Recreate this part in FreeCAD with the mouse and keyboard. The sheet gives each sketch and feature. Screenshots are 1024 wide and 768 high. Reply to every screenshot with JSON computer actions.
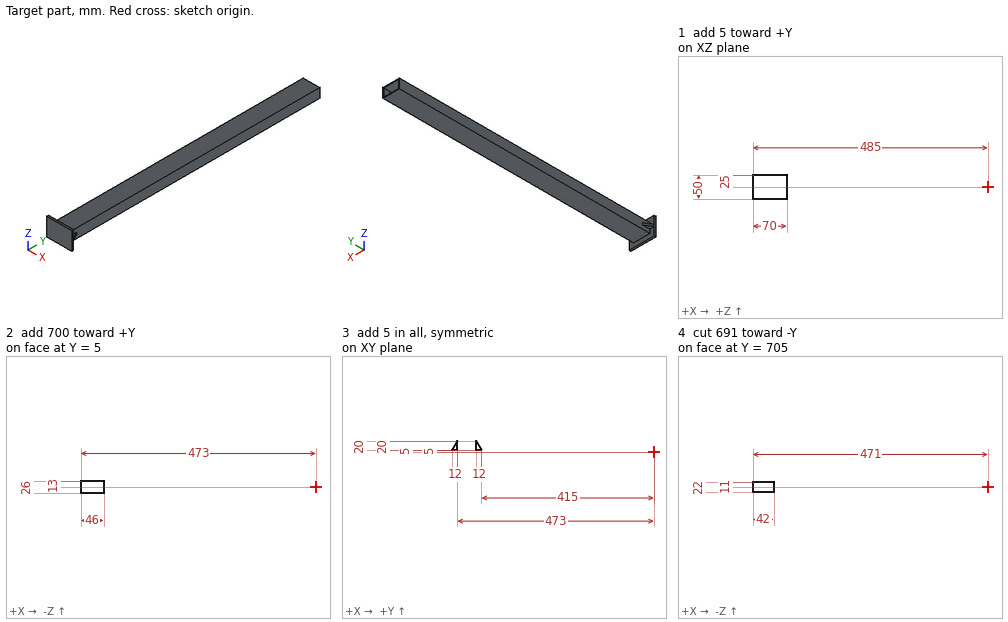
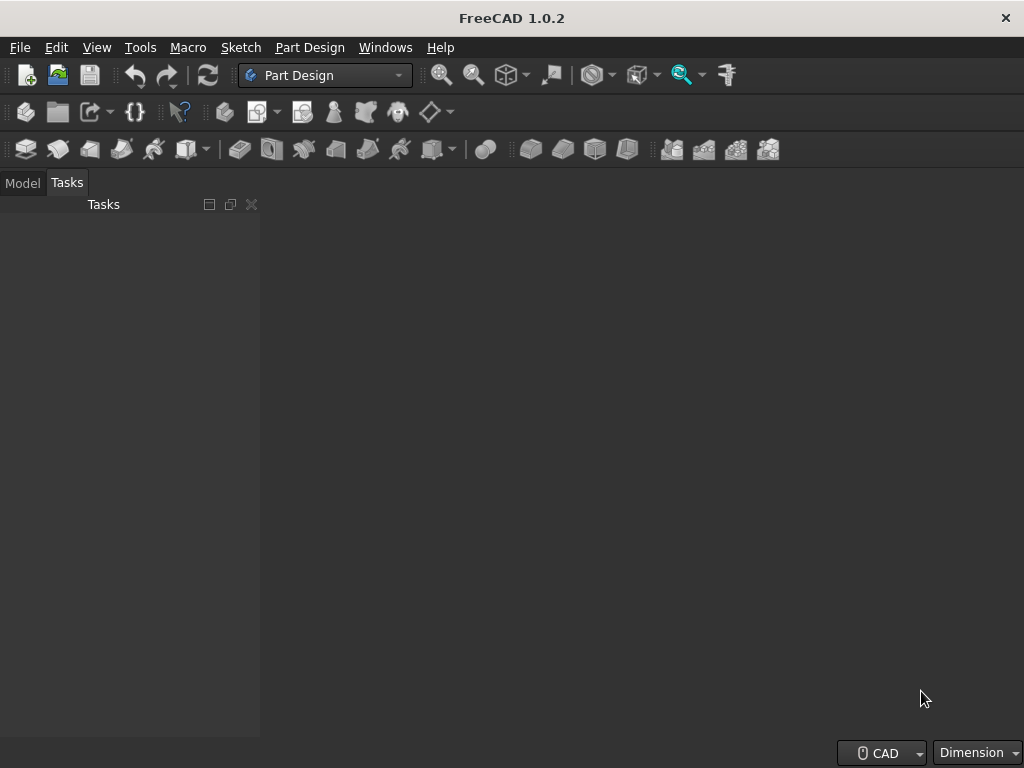
{"action": "left_click", "coordinate": [26, 76]}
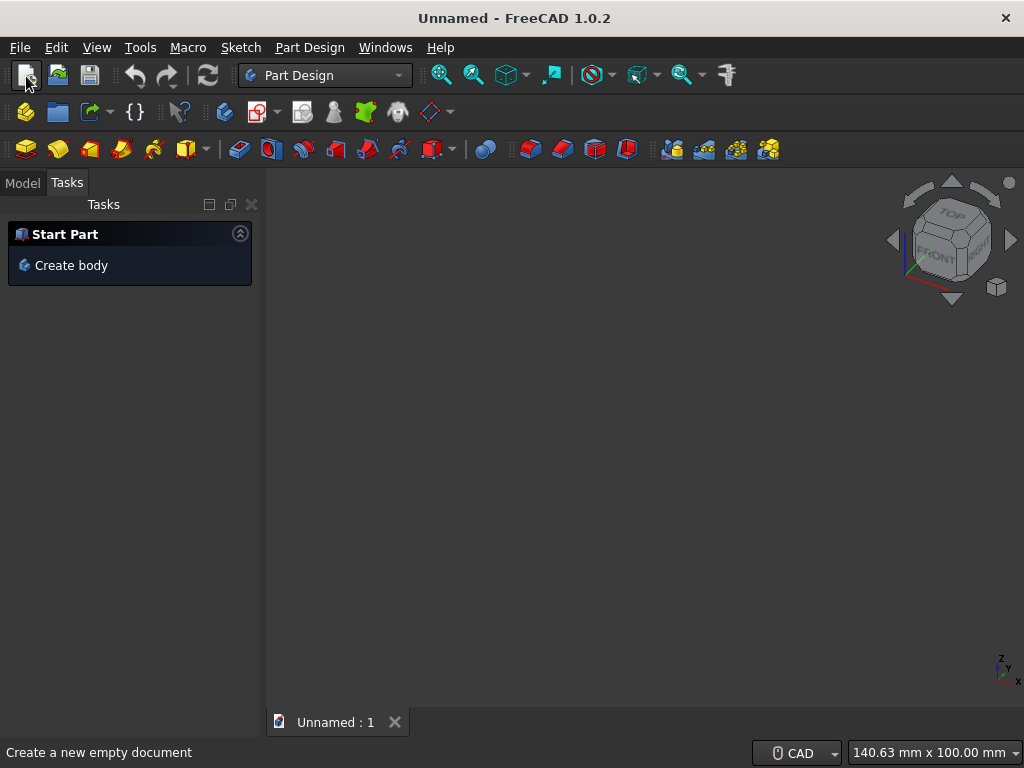
{"action": "left_click", "coordinate": [258, 112]}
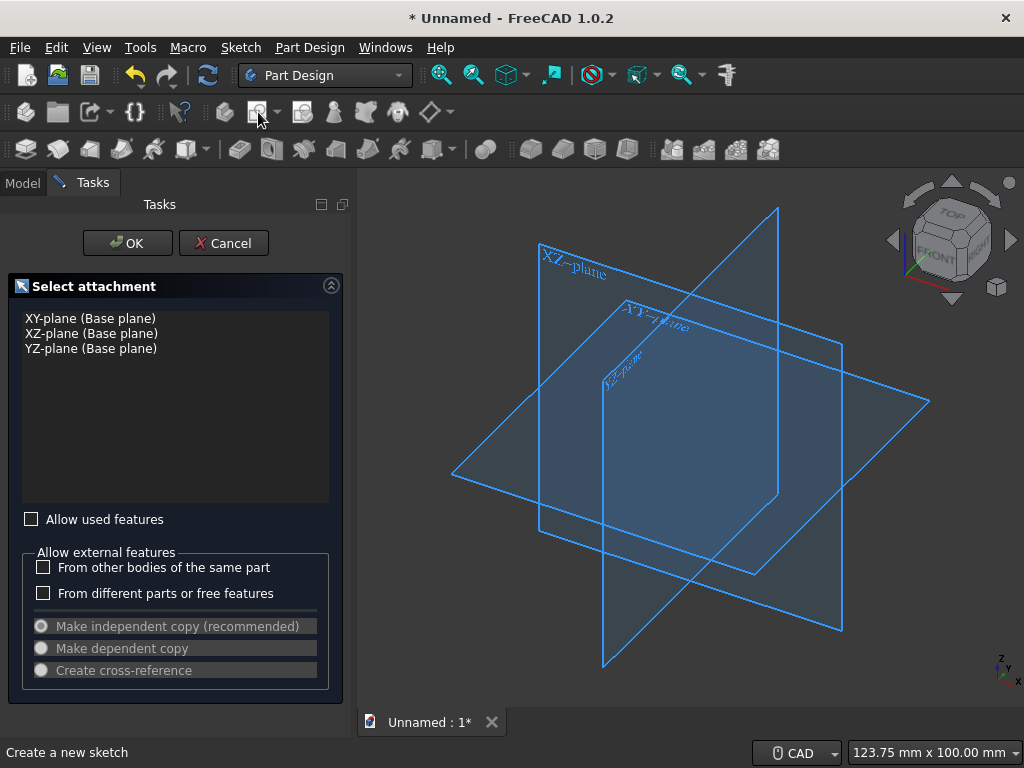
{"action": "left_click", "coordinate": [82, 334]}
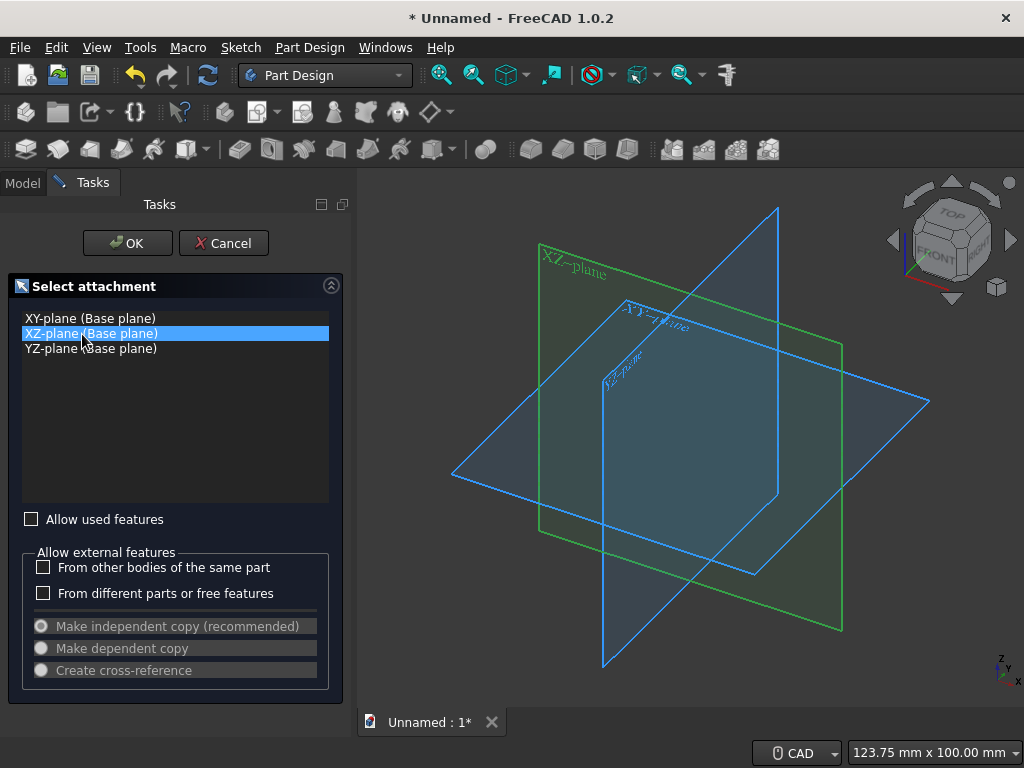
{"action": "left_click", "coordinate": [128, 243]}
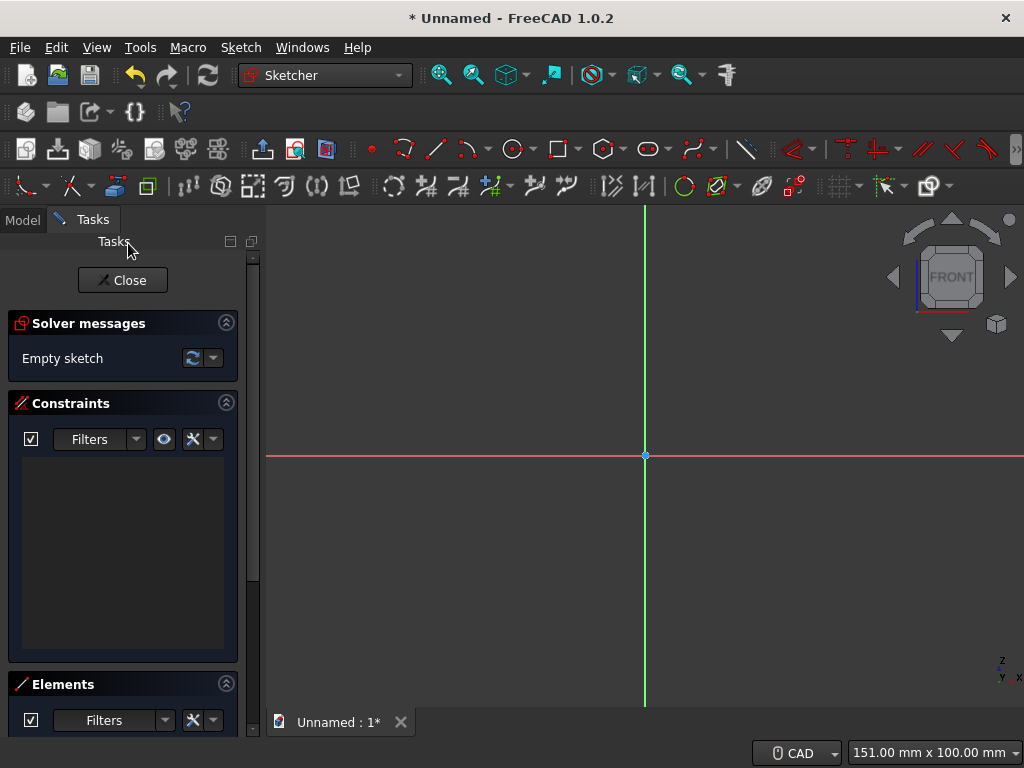
{"action": "scroll", "coordinate": [576, 456], "scroll_direction": "down", "scroll_amount": 5}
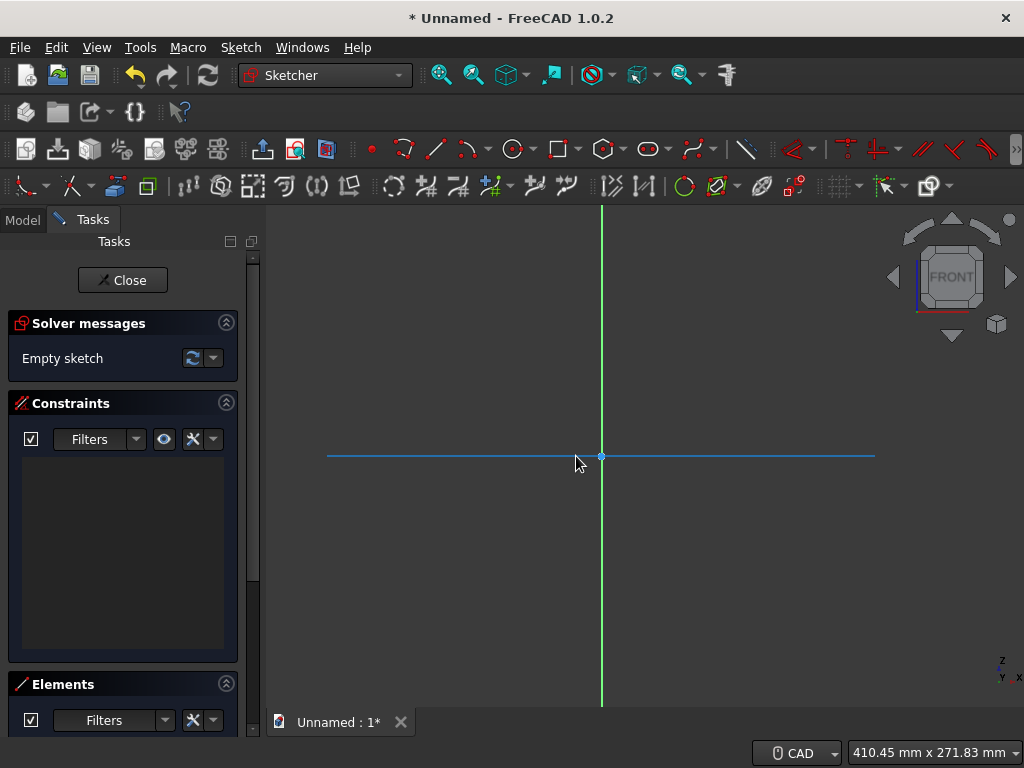
{"action": "scroll", "coordinate": [576, 456], "scroll_direction": "down", "scroll_amount": 5}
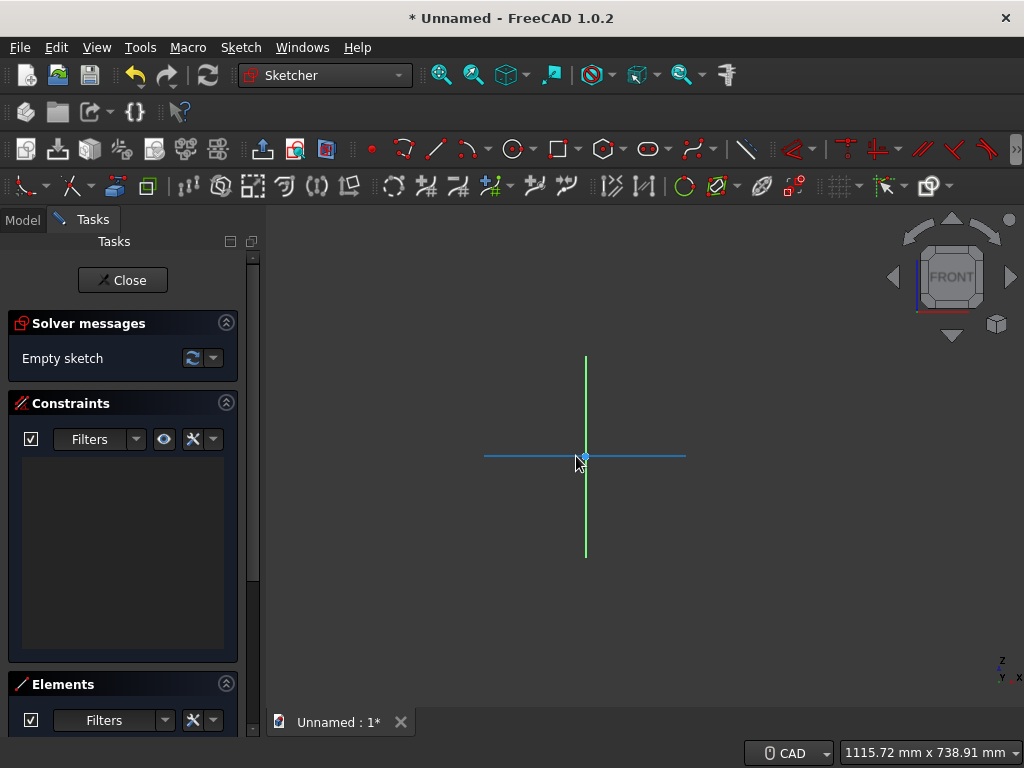
{"action": "scroll", "coordinate": [576, 456], "scroll_direction": "down", "scroll_amount": 5}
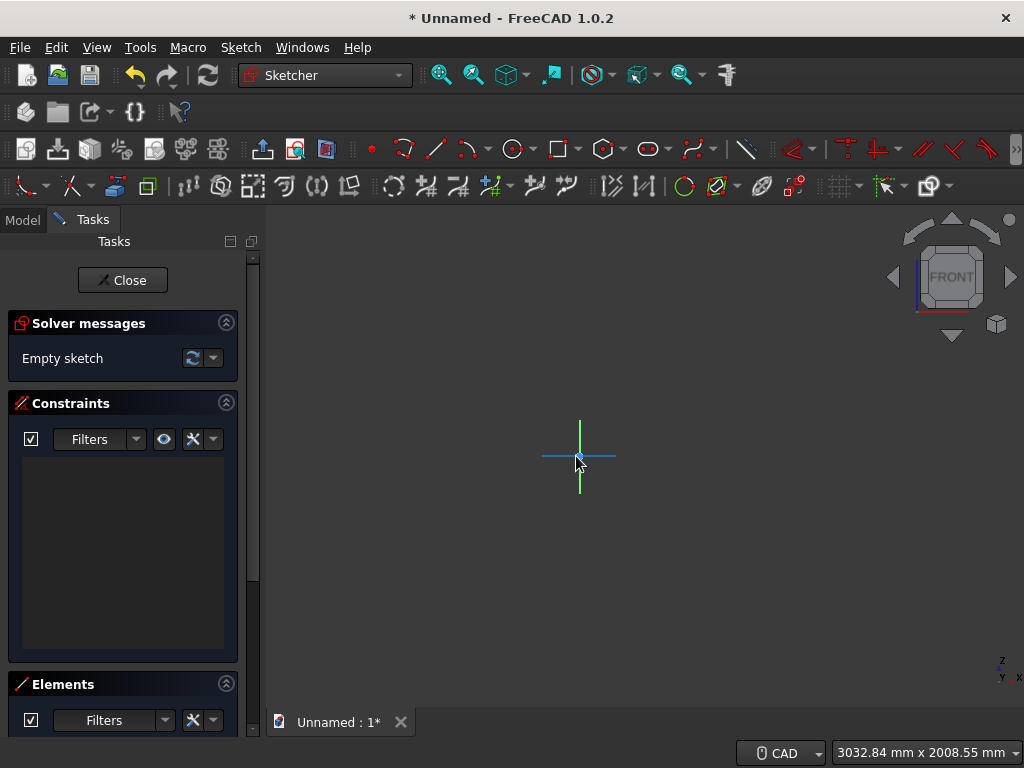
{"action": "scroll", "coordinate": [462, 457], "scroll_direction": "up", "scroll_amount": 15}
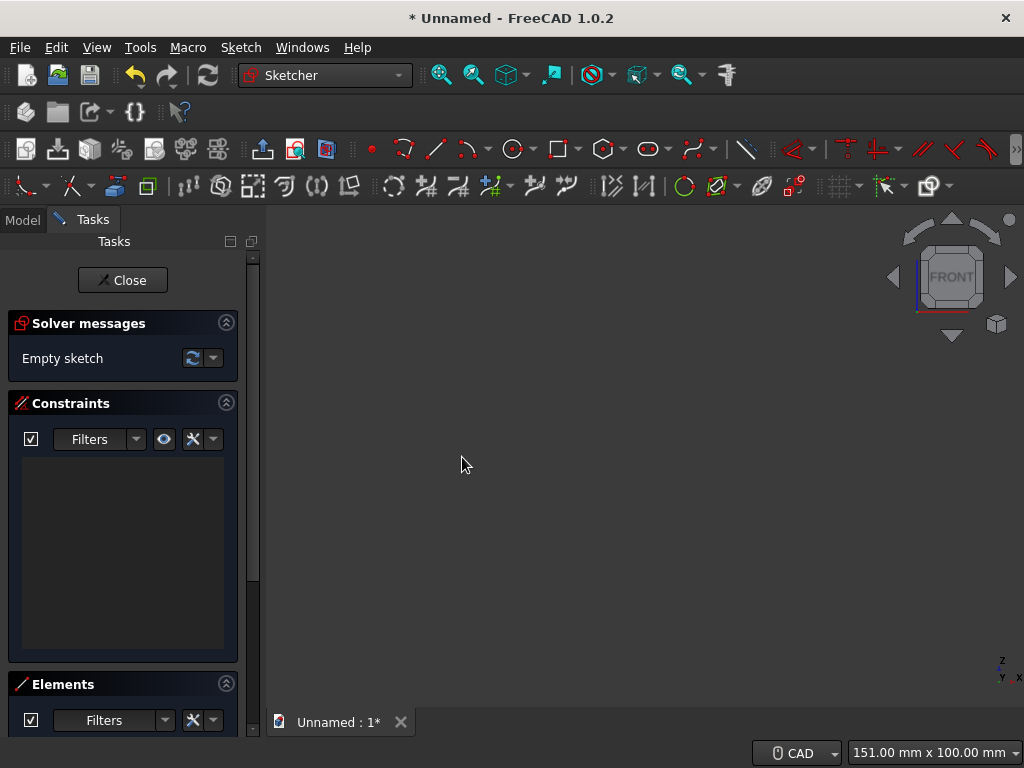
{"action": "left_click", "coordinate": [558, 150]}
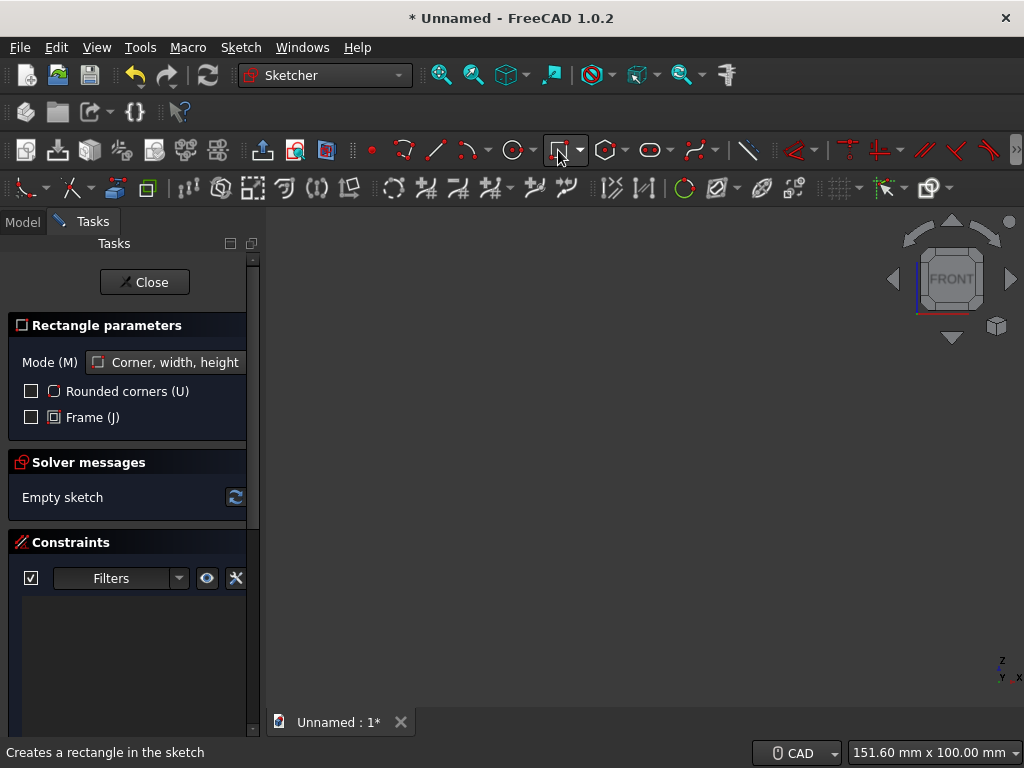
{"action": "left_click", "coordinate": [390, 313]}
{"action": "left_click", "coordinate": [740, 563]}
{"action": "key", "text": "Escape"}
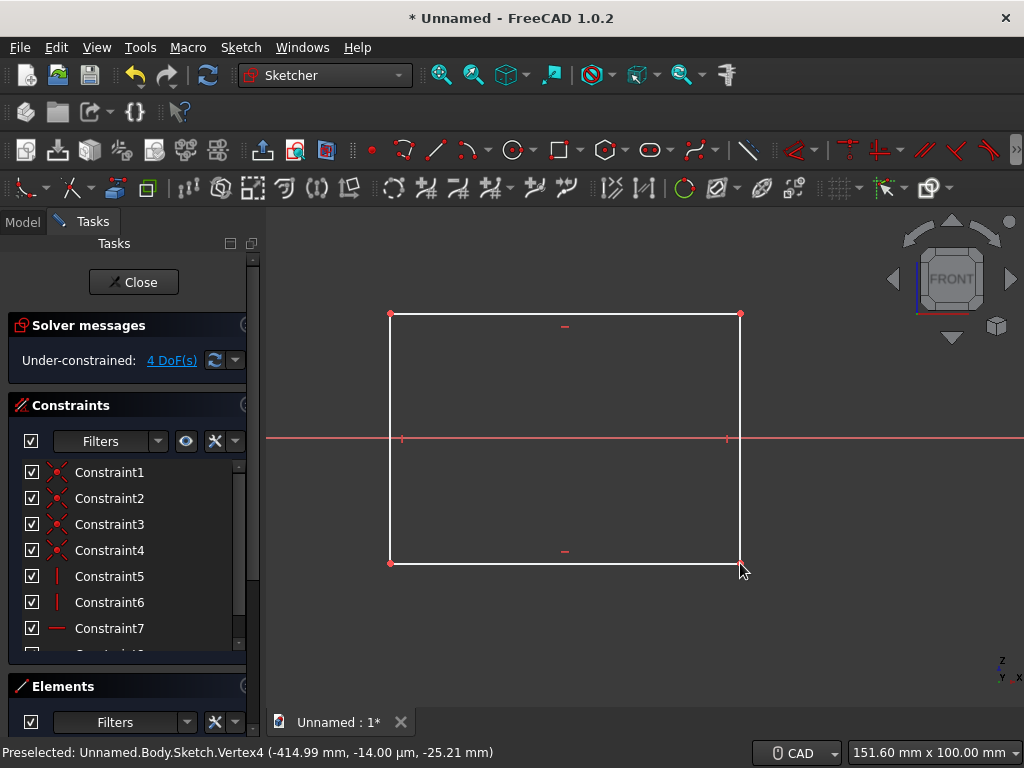
{"action": "left_click", "coordinate": [390, 389]}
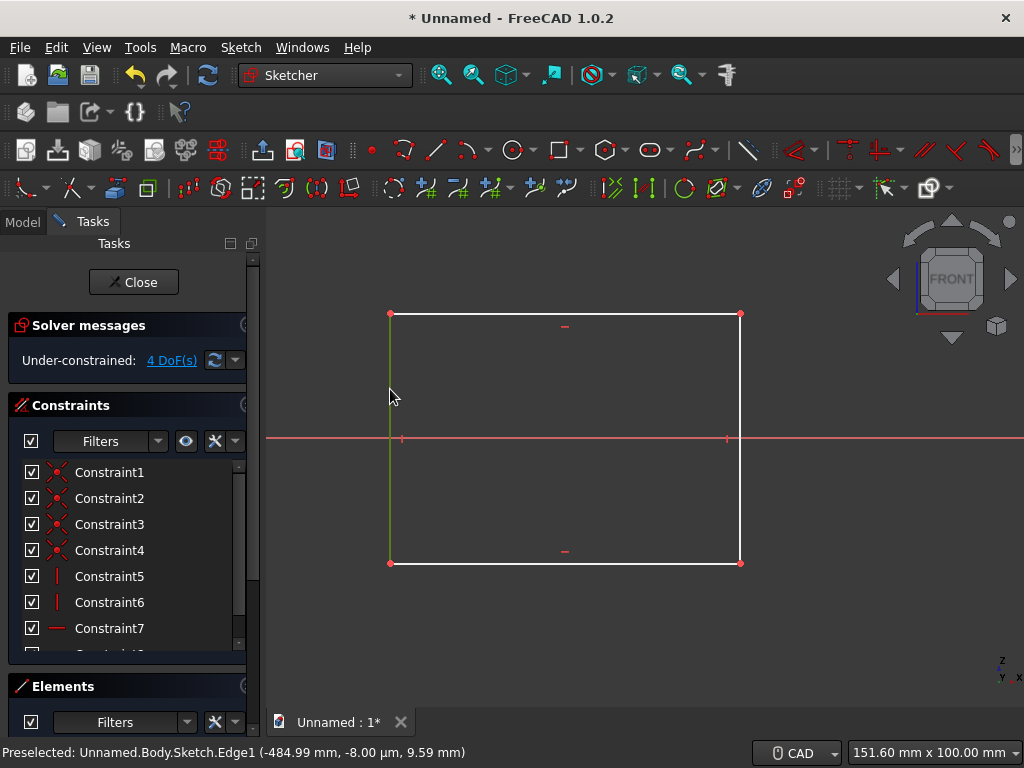
{"action": "left_click", "coordinate": [816, 150]}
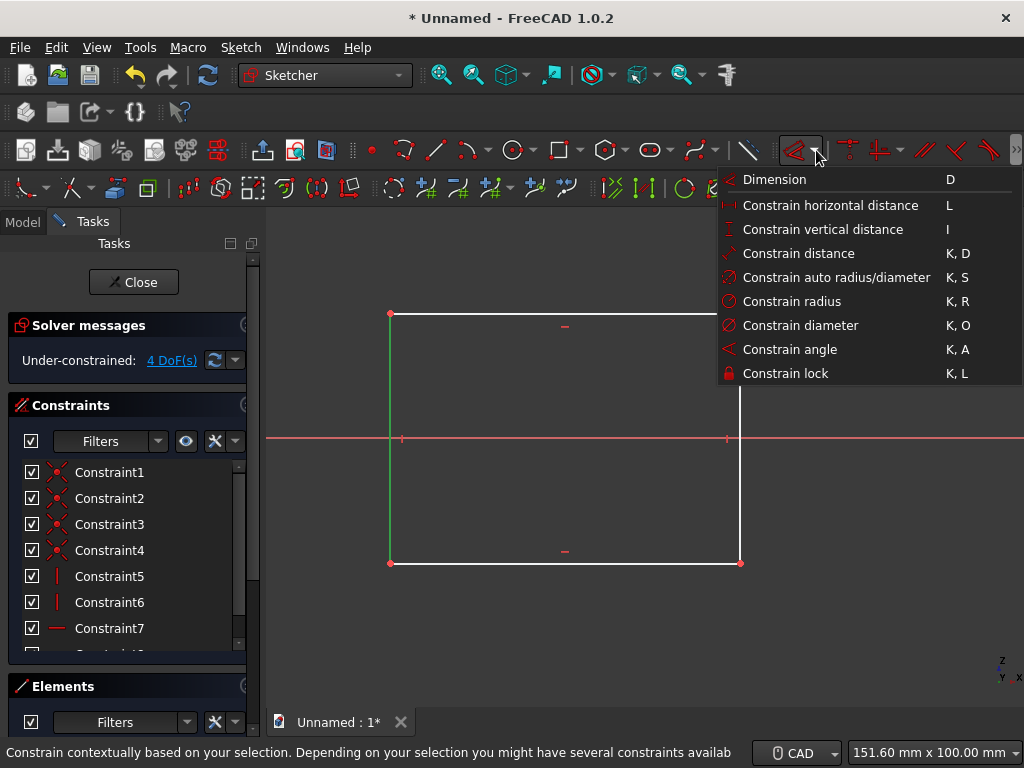
{"action": "left_click", "coordinate": [870, 229]}